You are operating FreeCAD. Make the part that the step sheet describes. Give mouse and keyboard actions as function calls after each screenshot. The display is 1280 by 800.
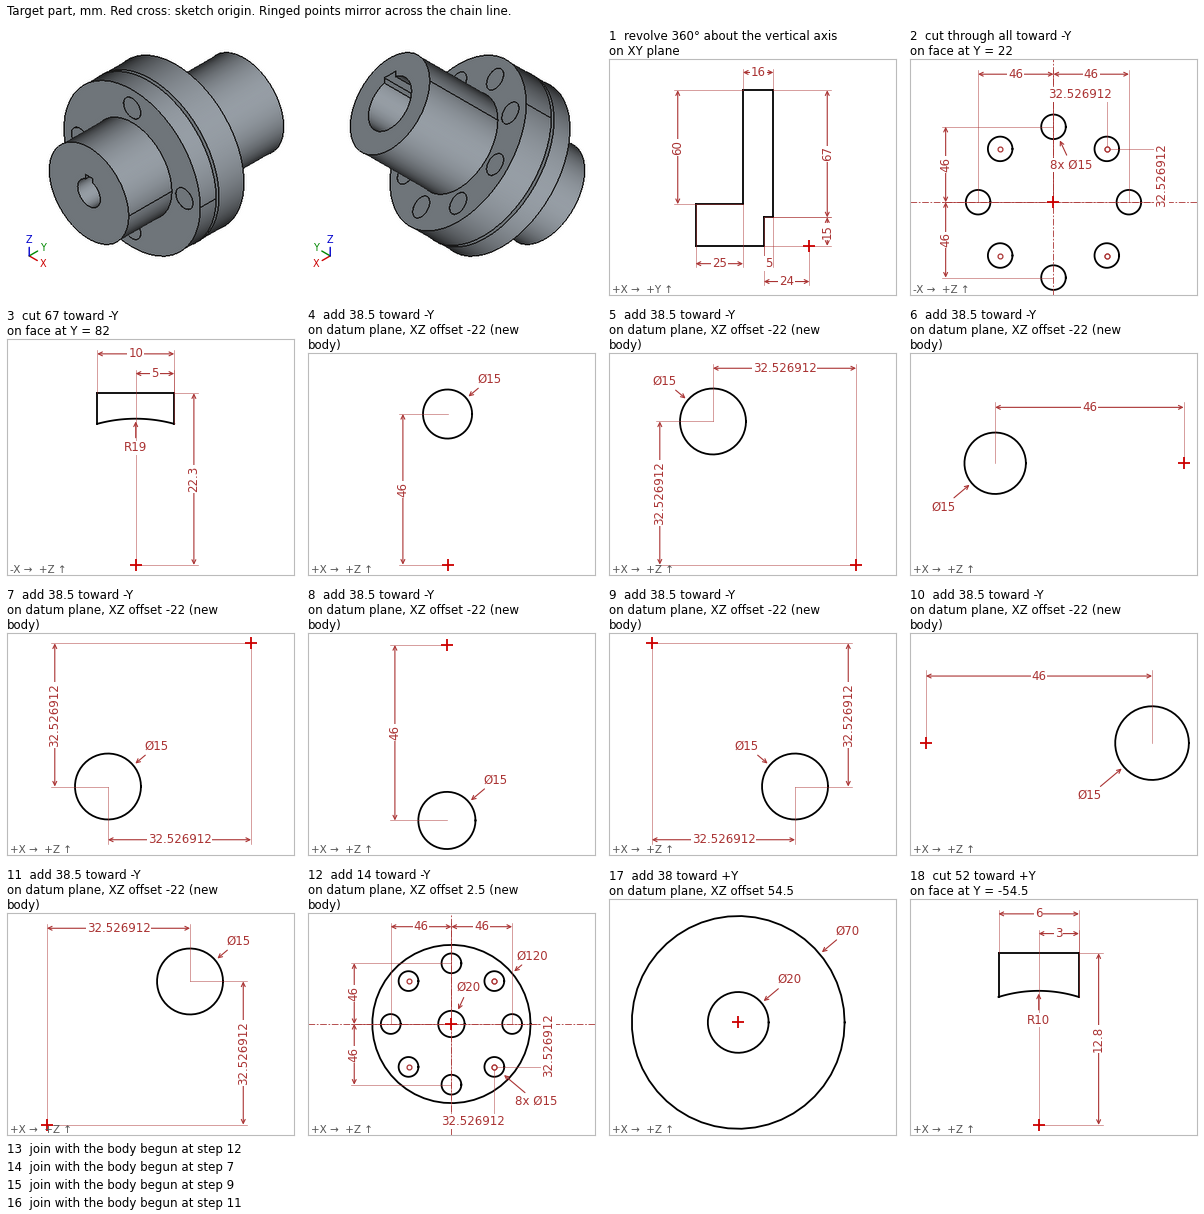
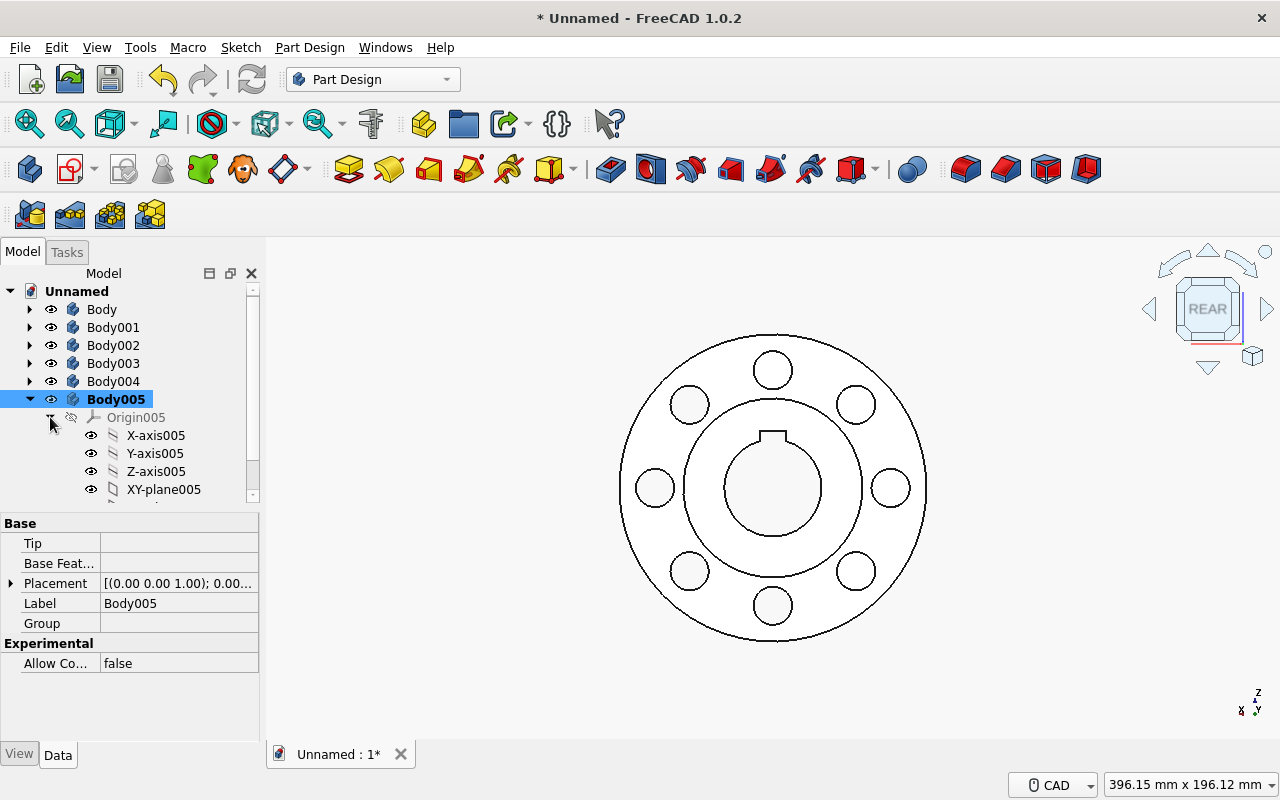
scroll(100, 395, down, 3)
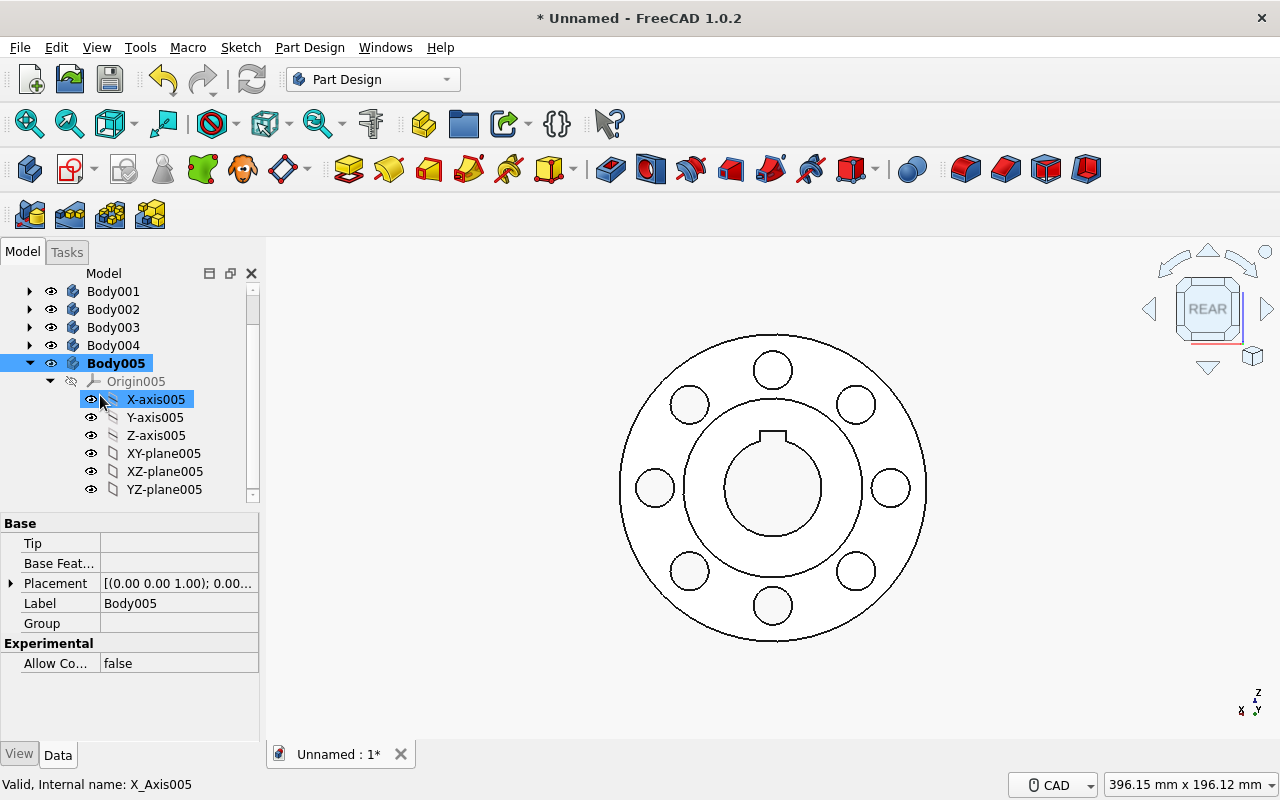
click(136, 471)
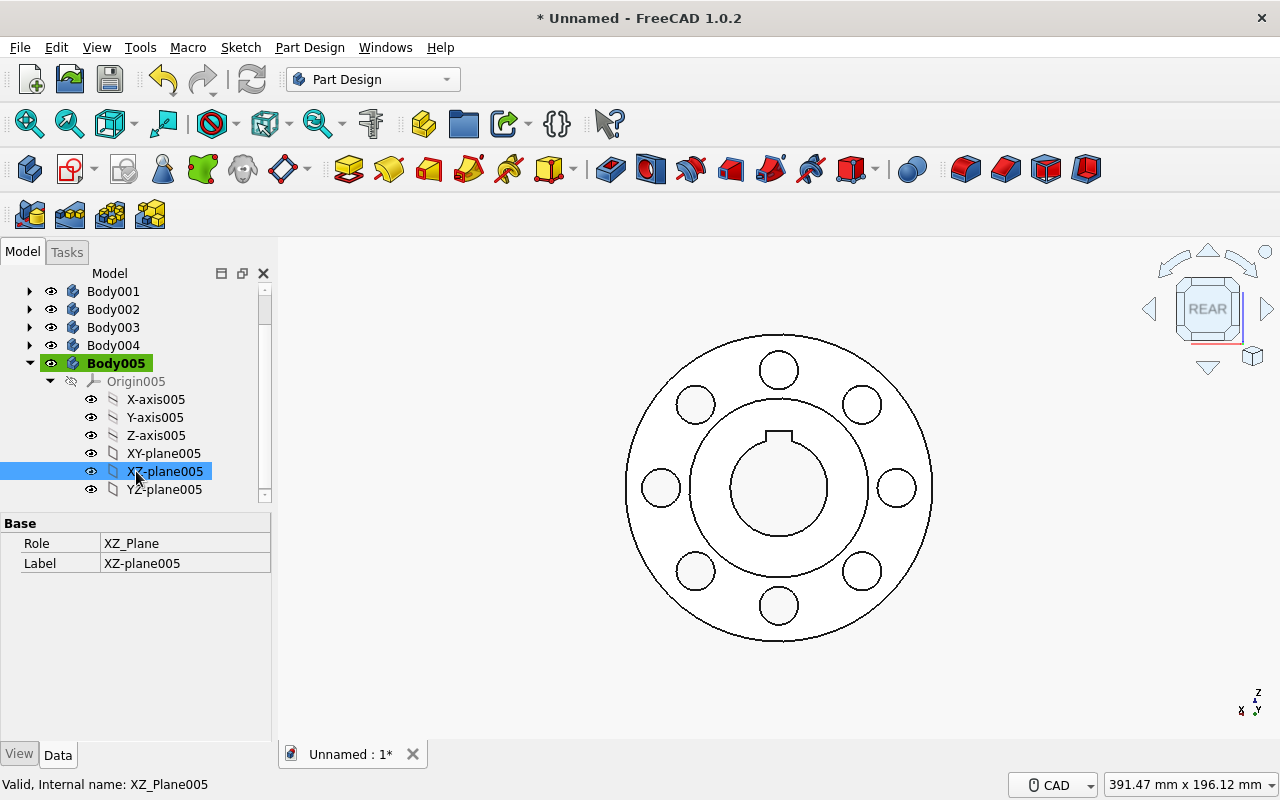
click(284, 170)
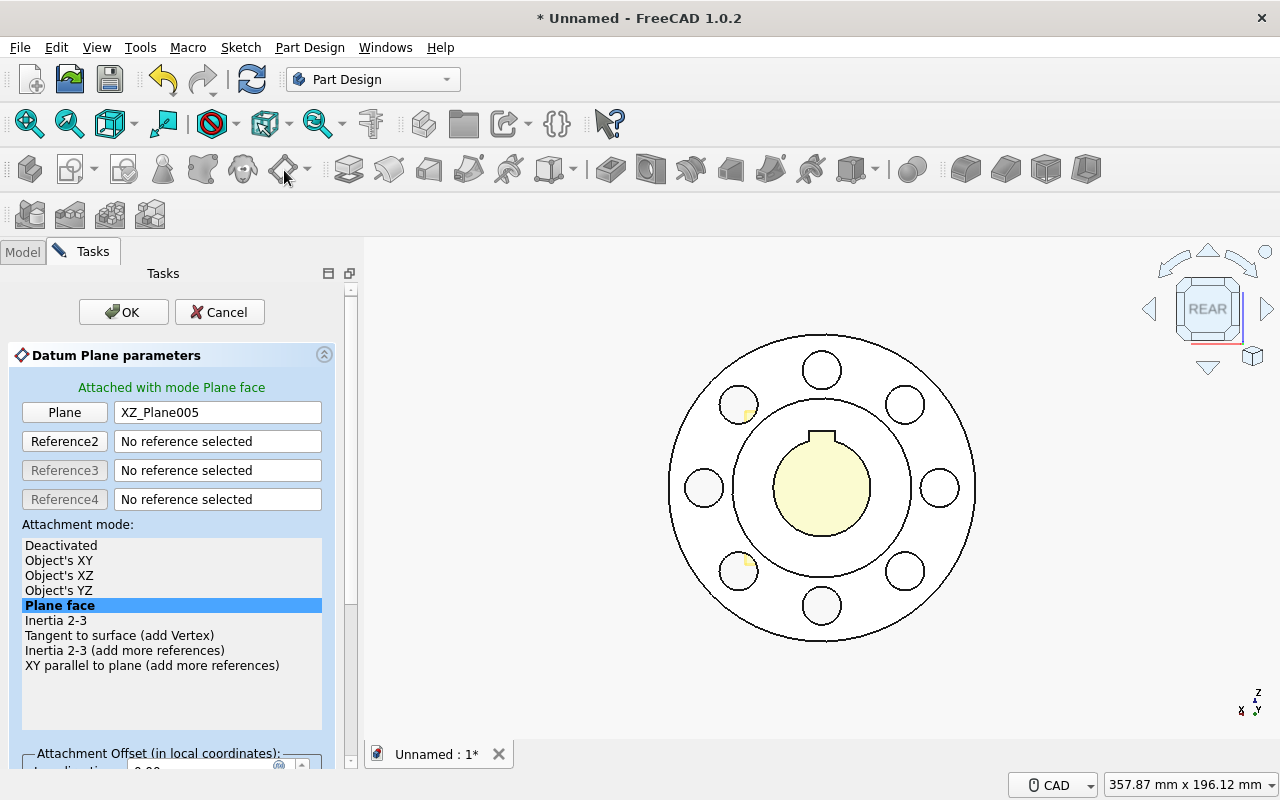
scroll(351, 526, down, 3)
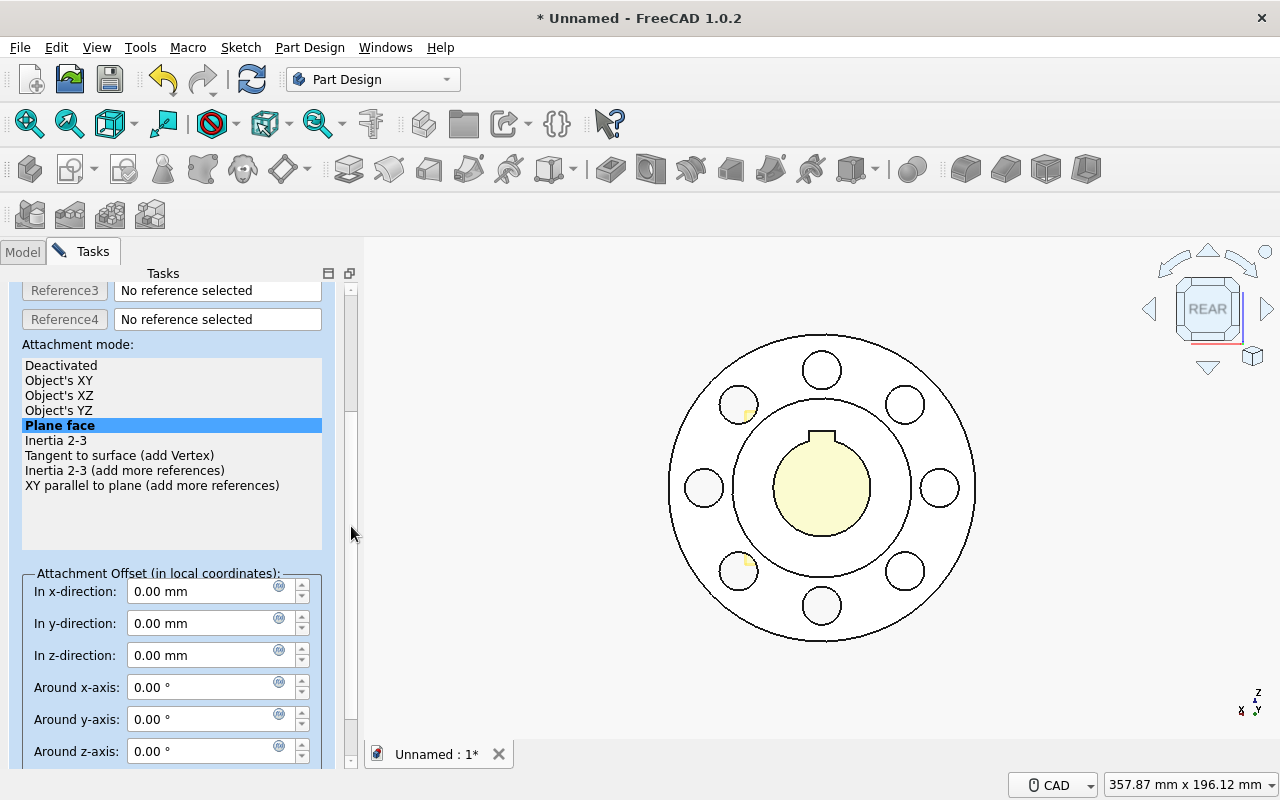
triple_click(210, 655)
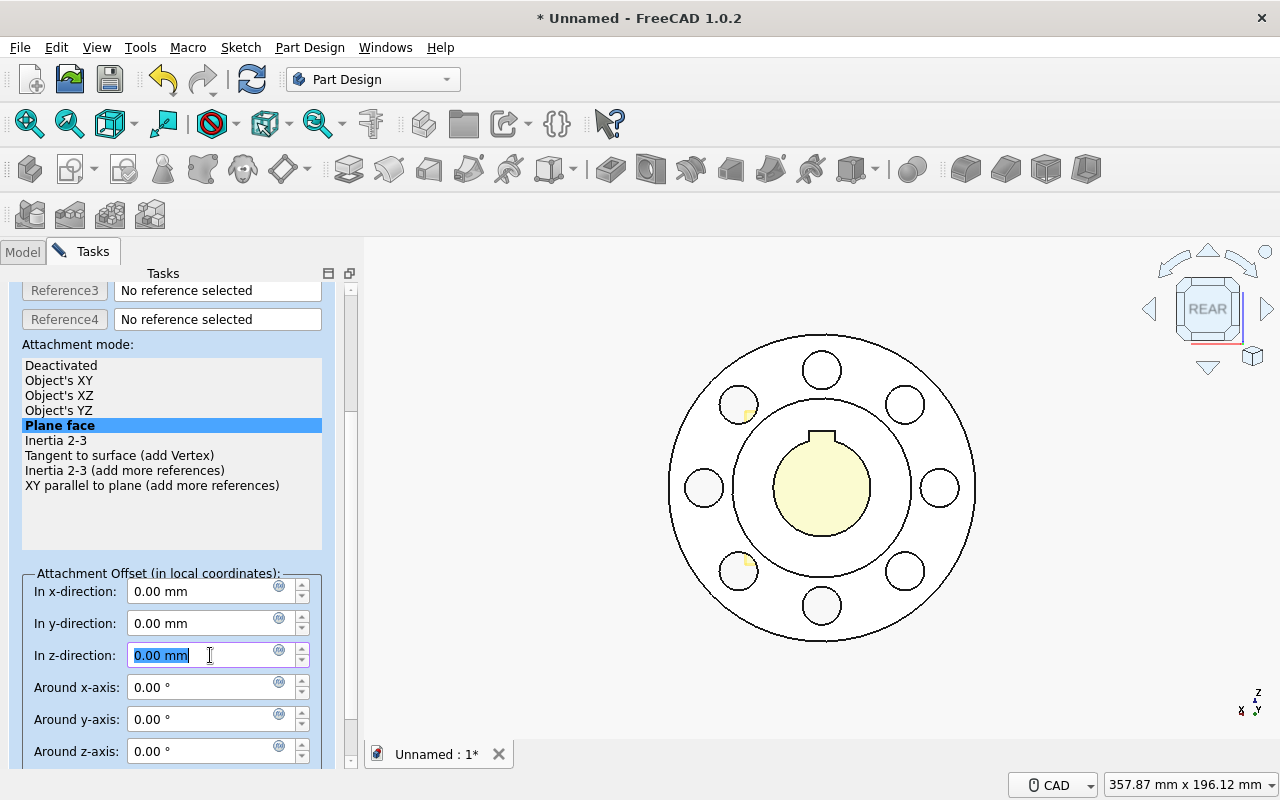
text(-22)
key(Tab)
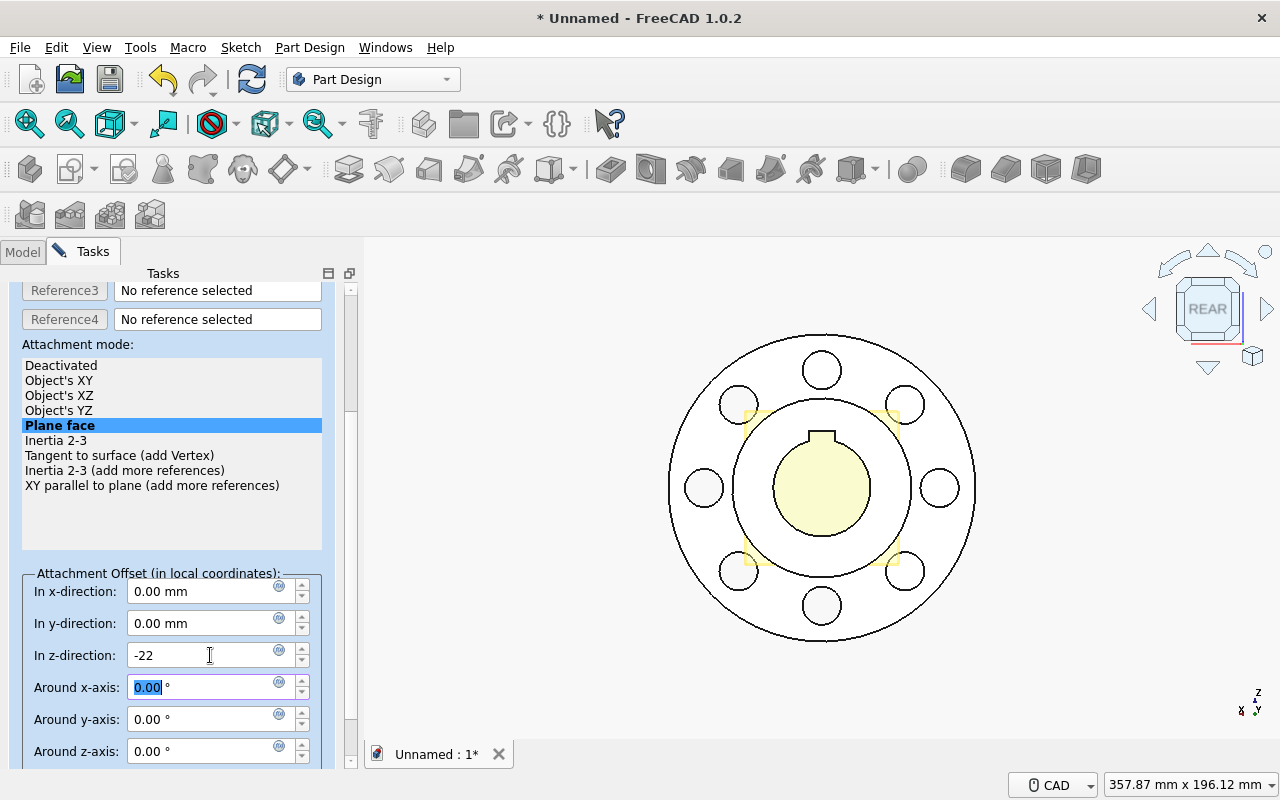
scroll(351, 526, up, 4)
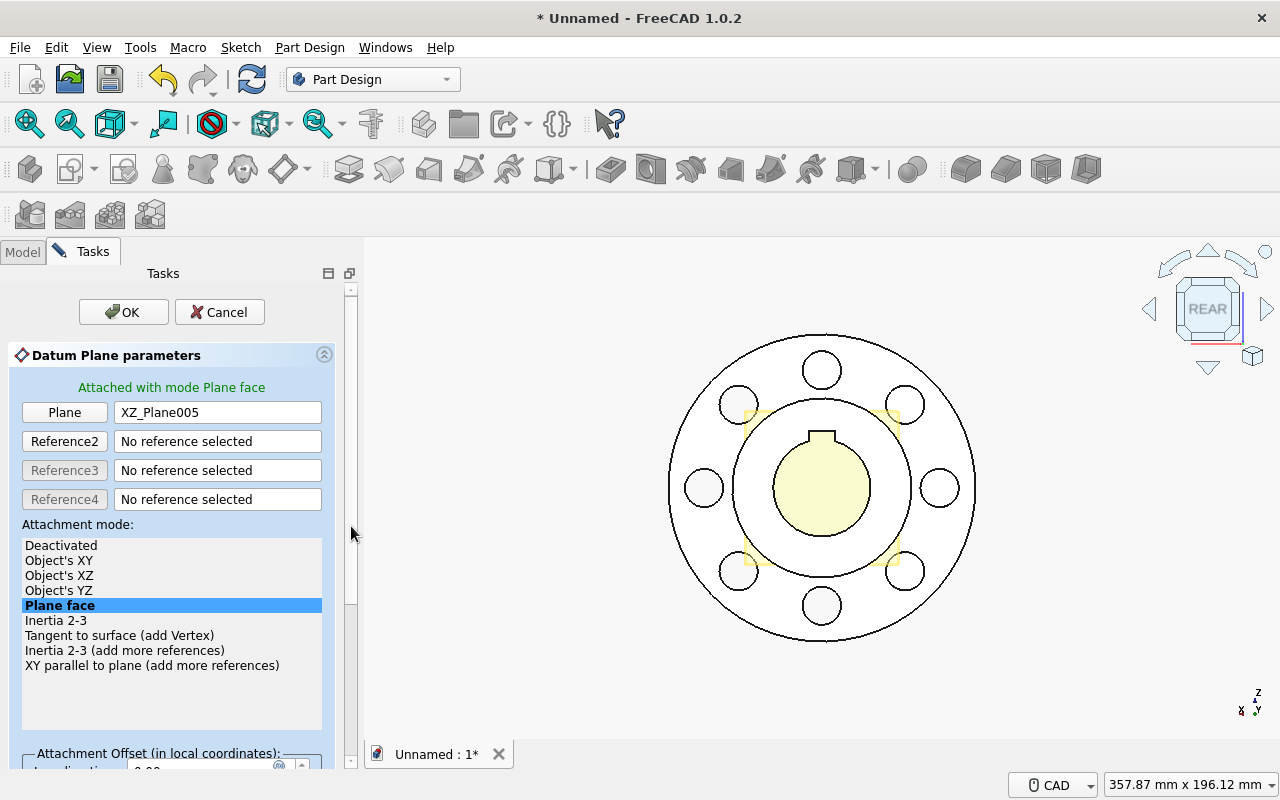
click(124, 312)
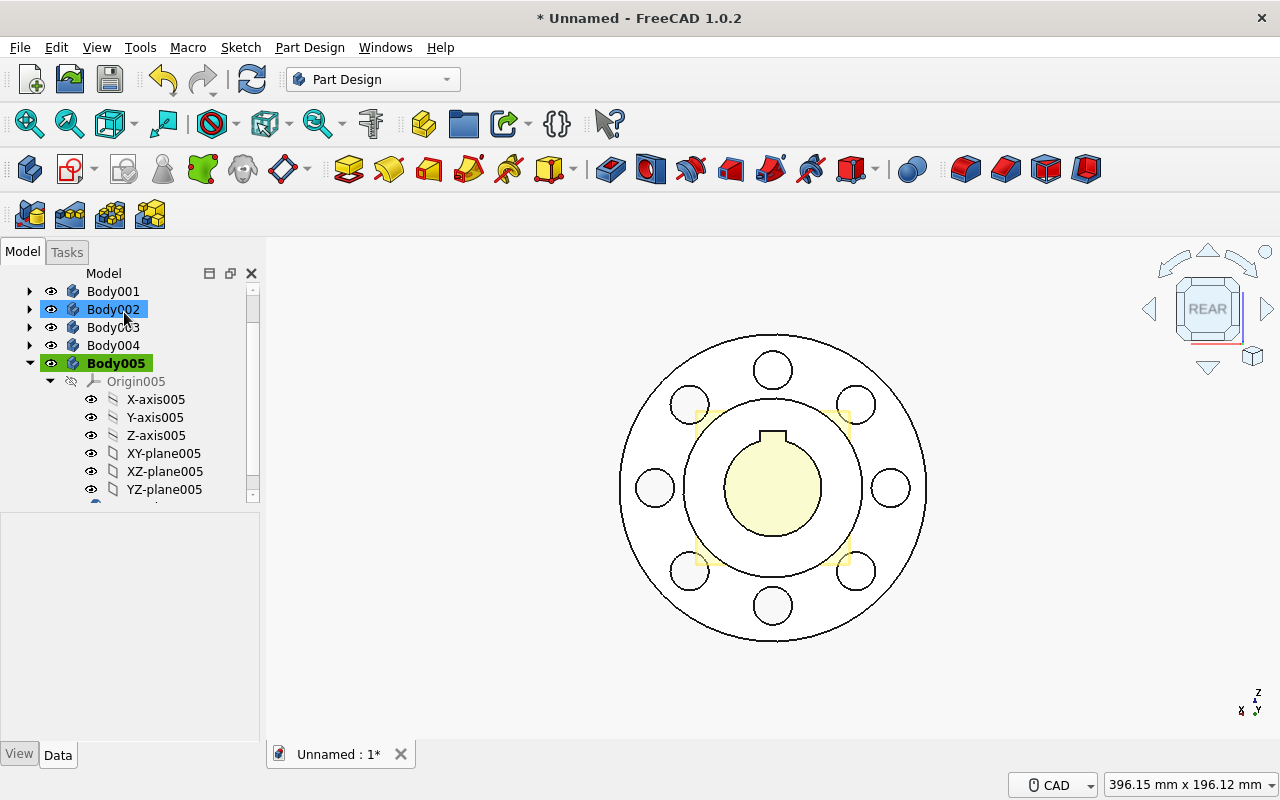
scroll(120, 395, down, 3)